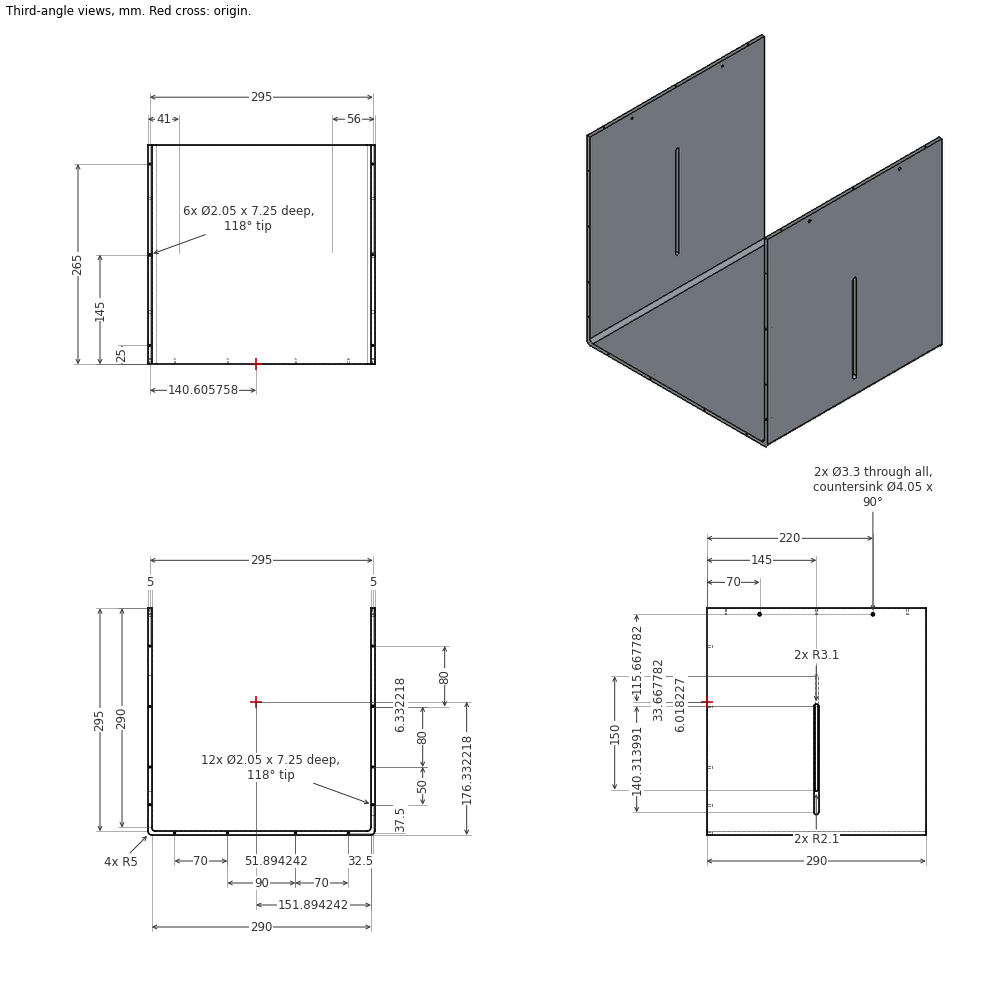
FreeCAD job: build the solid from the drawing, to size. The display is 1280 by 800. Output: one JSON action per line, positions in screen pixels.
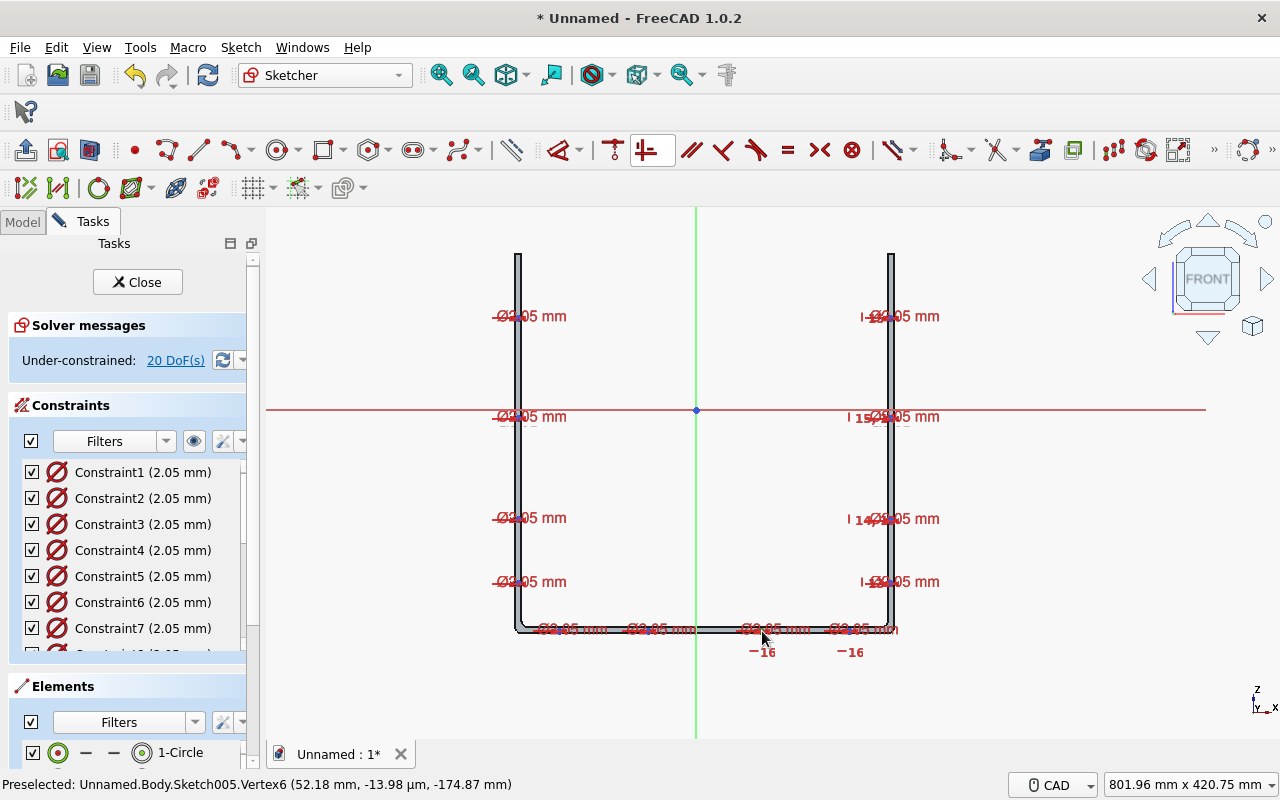
{"action": "left_click", "coordinate": [648, 631]}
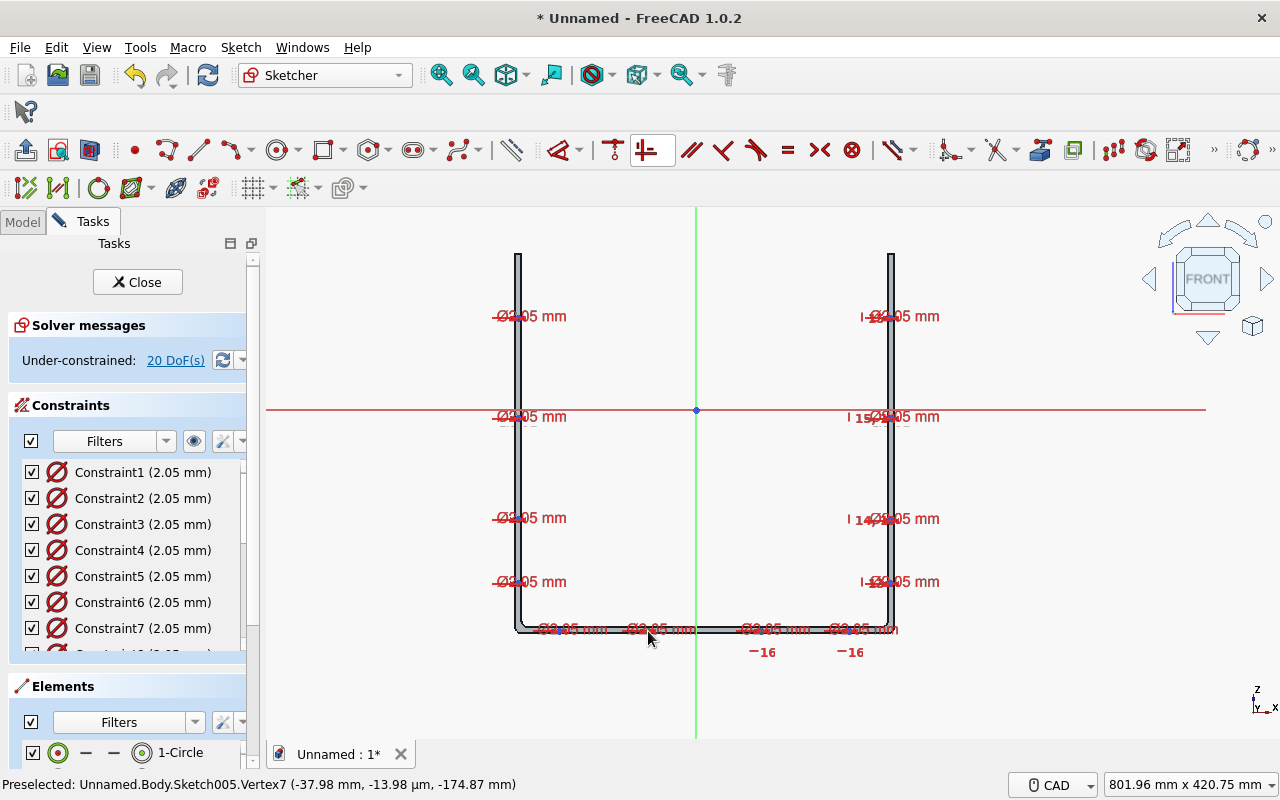
{"action": "left_click", "coordinate": [670, 150]}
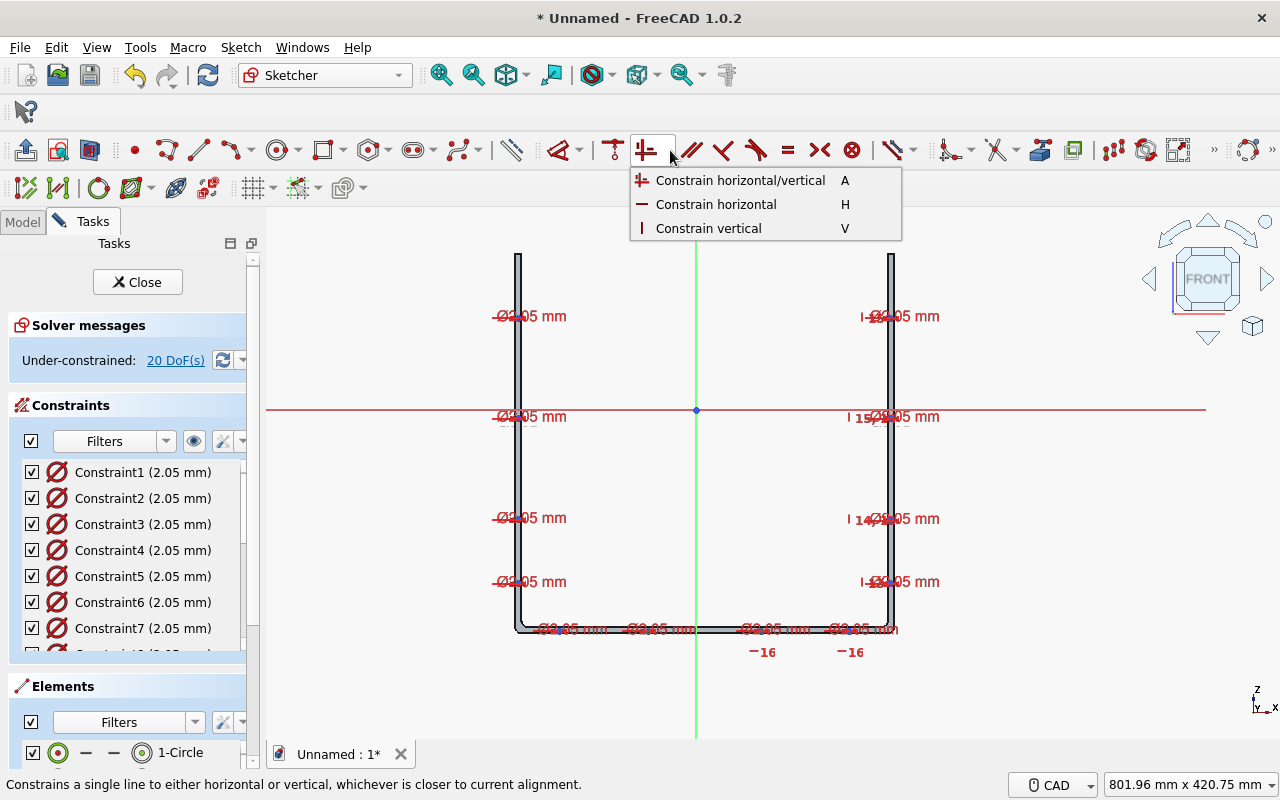
{"action": "left_click", "coordinate": [766, 204]}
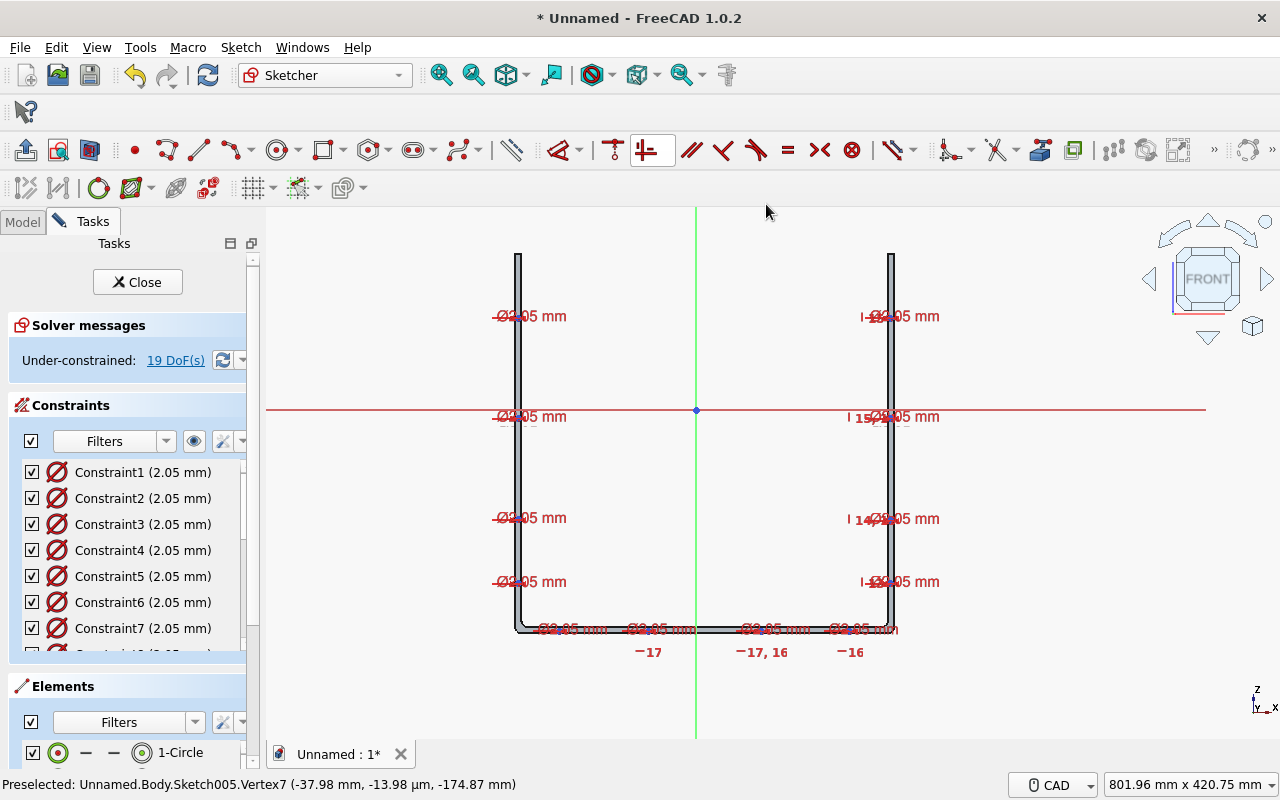
{"action": "left_click", "coordinate": [648, 631]}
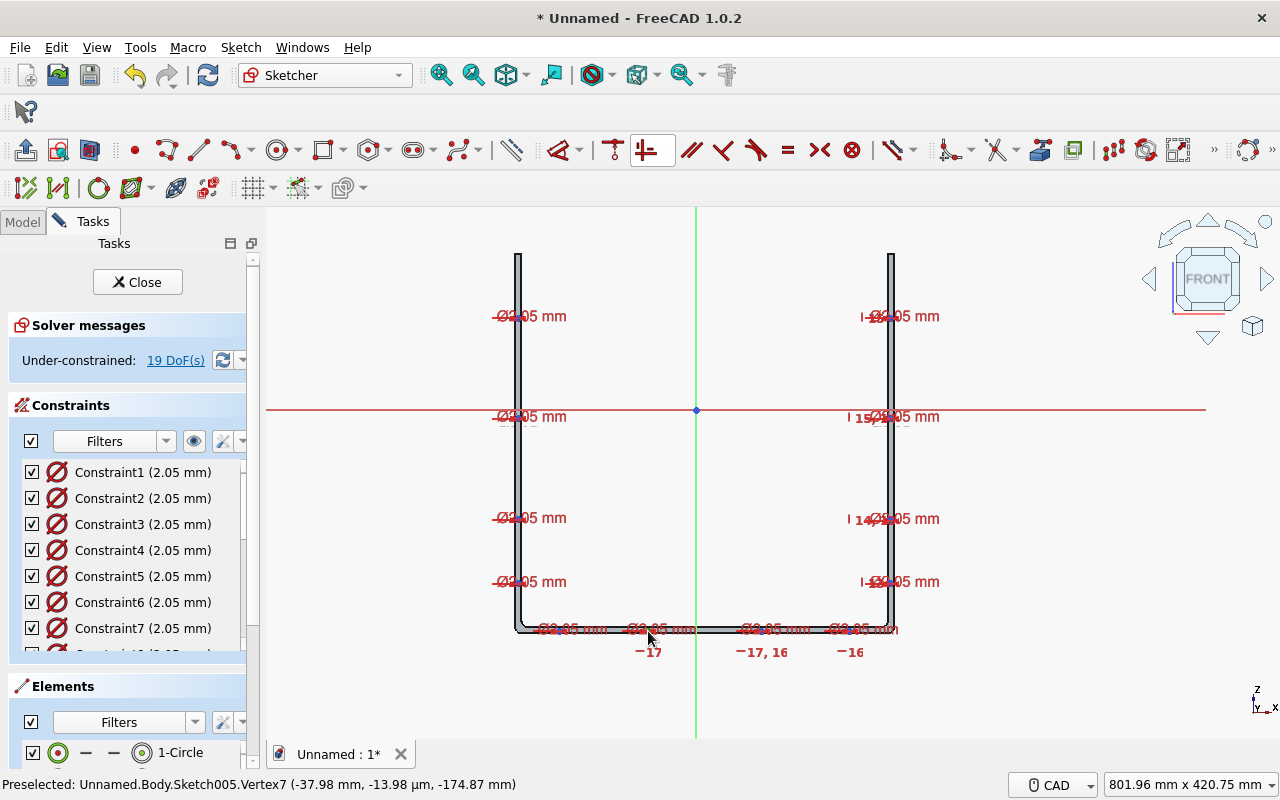
{"action": "left_click", "coordinate": [559, 631]}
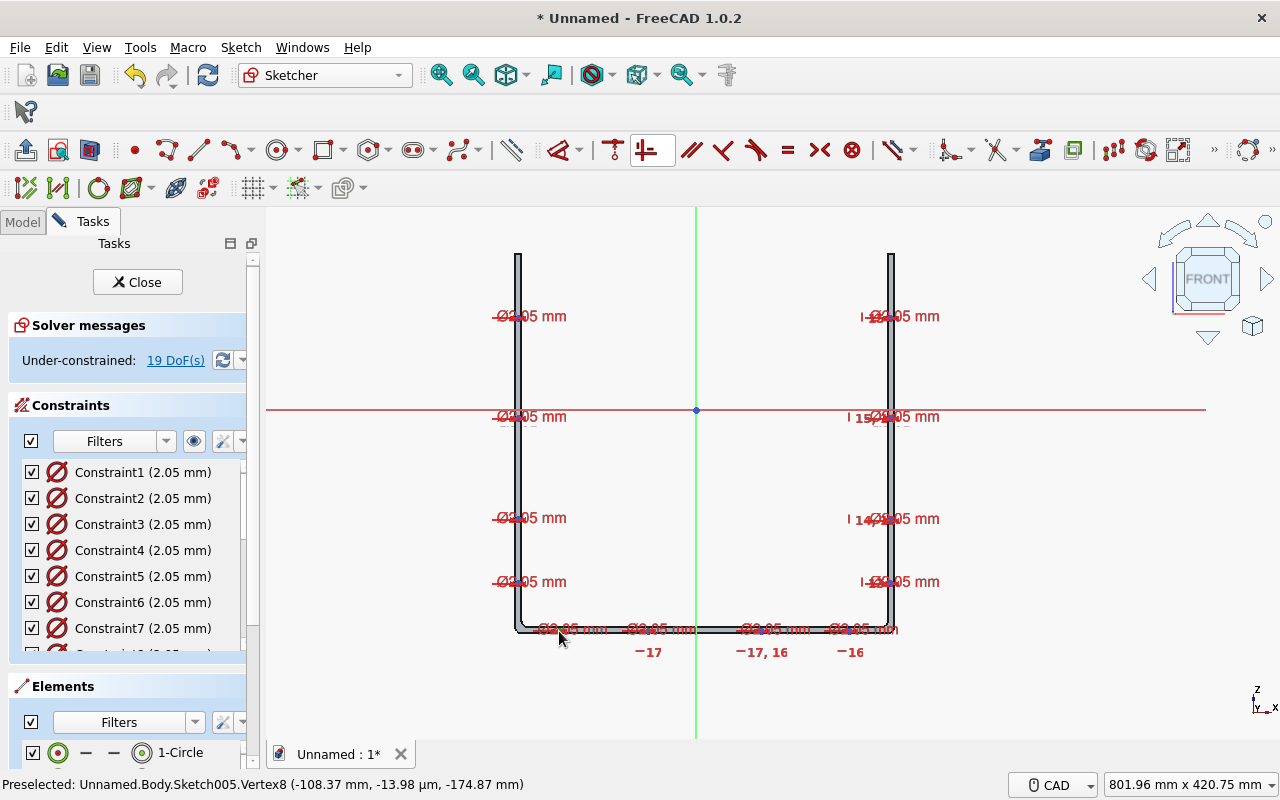
{"action": "left_click", "coordinate": [670, 150]}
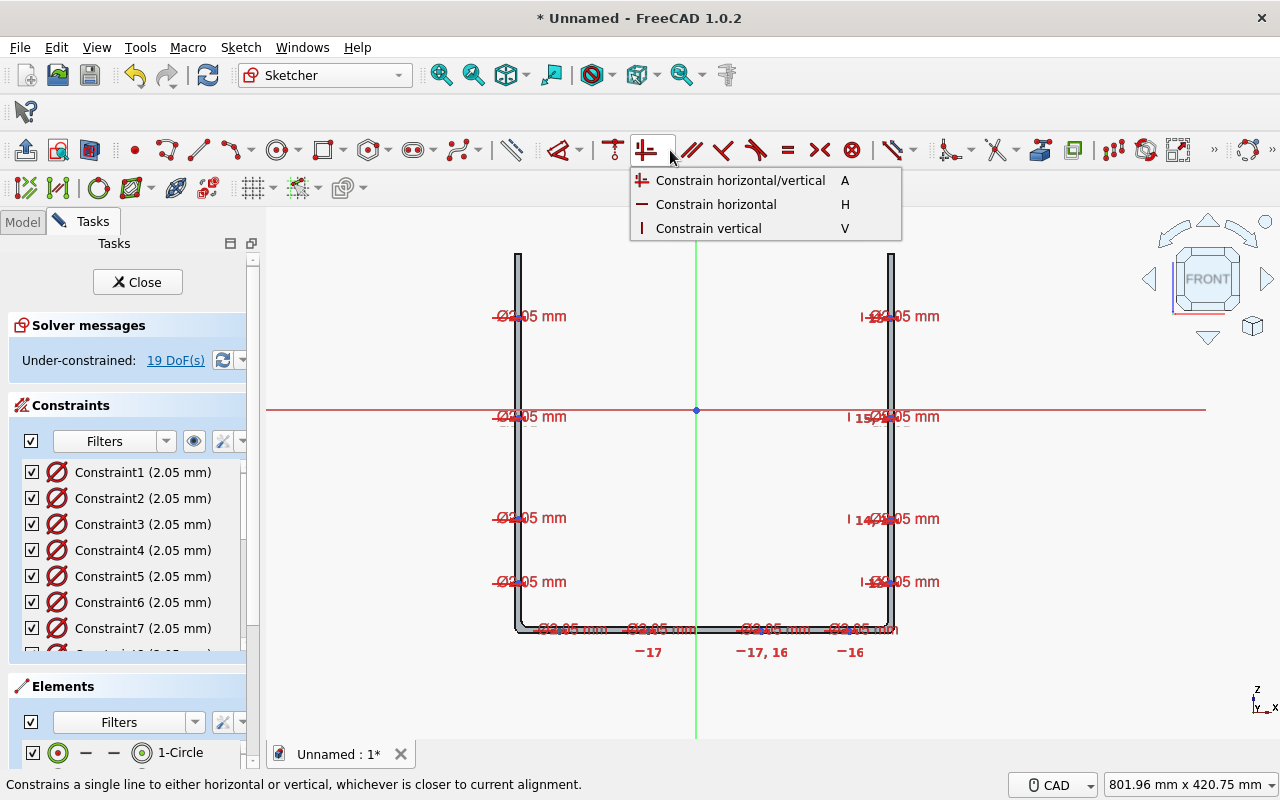
{"action": "left_click", "coordinate": [766, 204]}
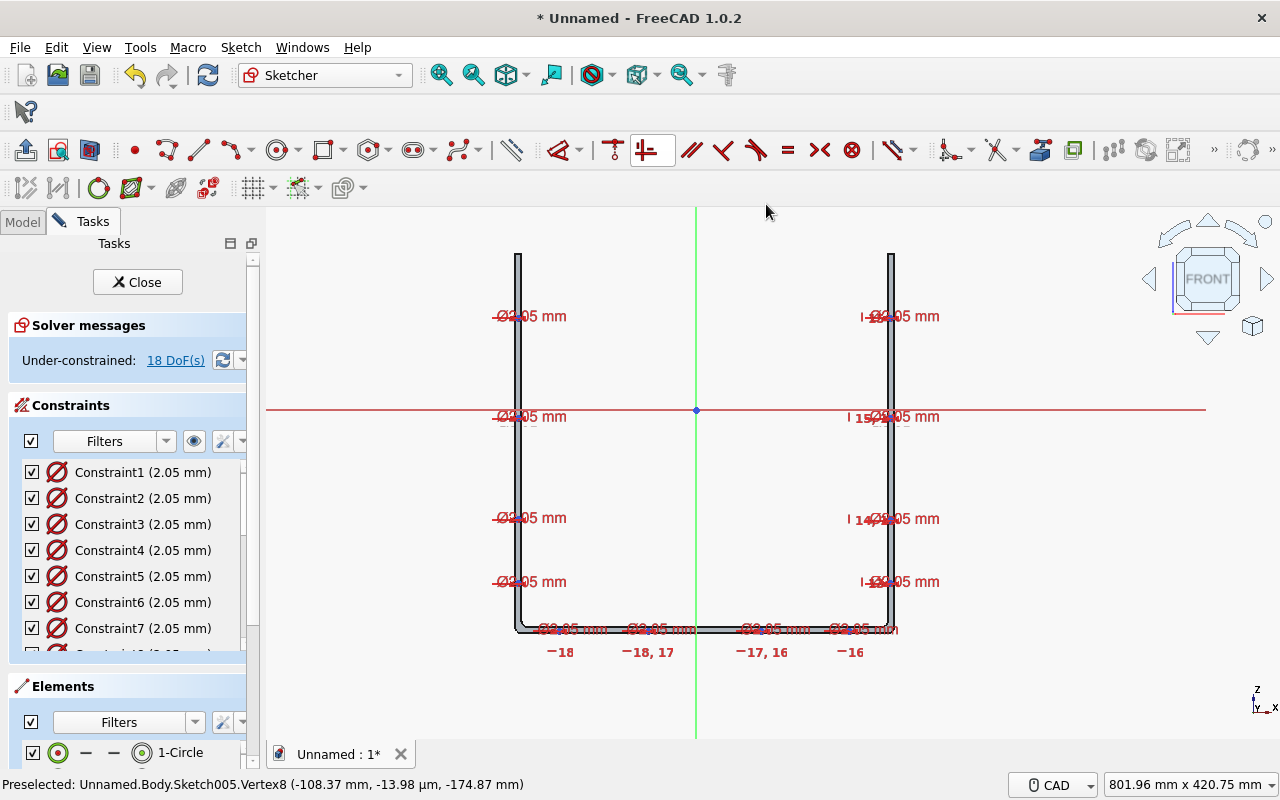
{"action": "left_click", "coordinate": [891, 318]}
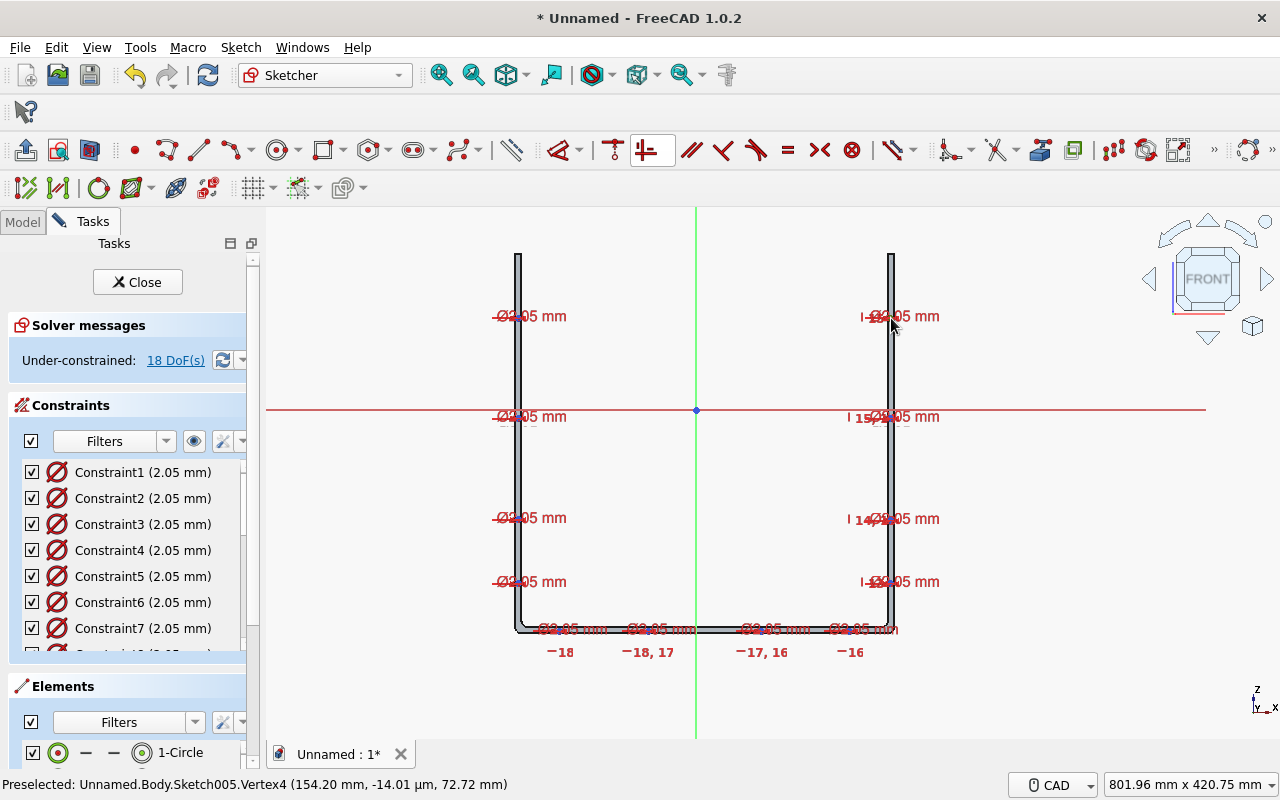
{"action": "left_click", "coordinate": [518, 318]}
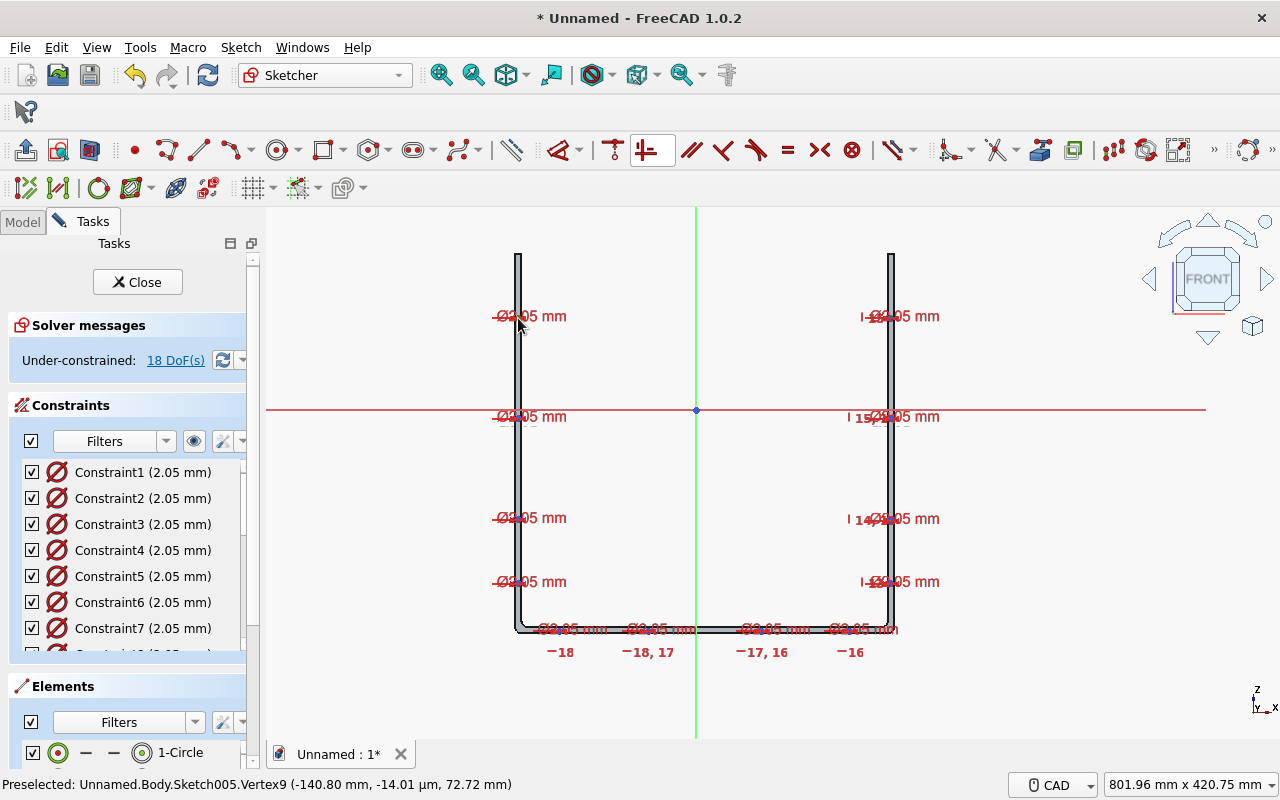
{"action": "key", "text": "h"}